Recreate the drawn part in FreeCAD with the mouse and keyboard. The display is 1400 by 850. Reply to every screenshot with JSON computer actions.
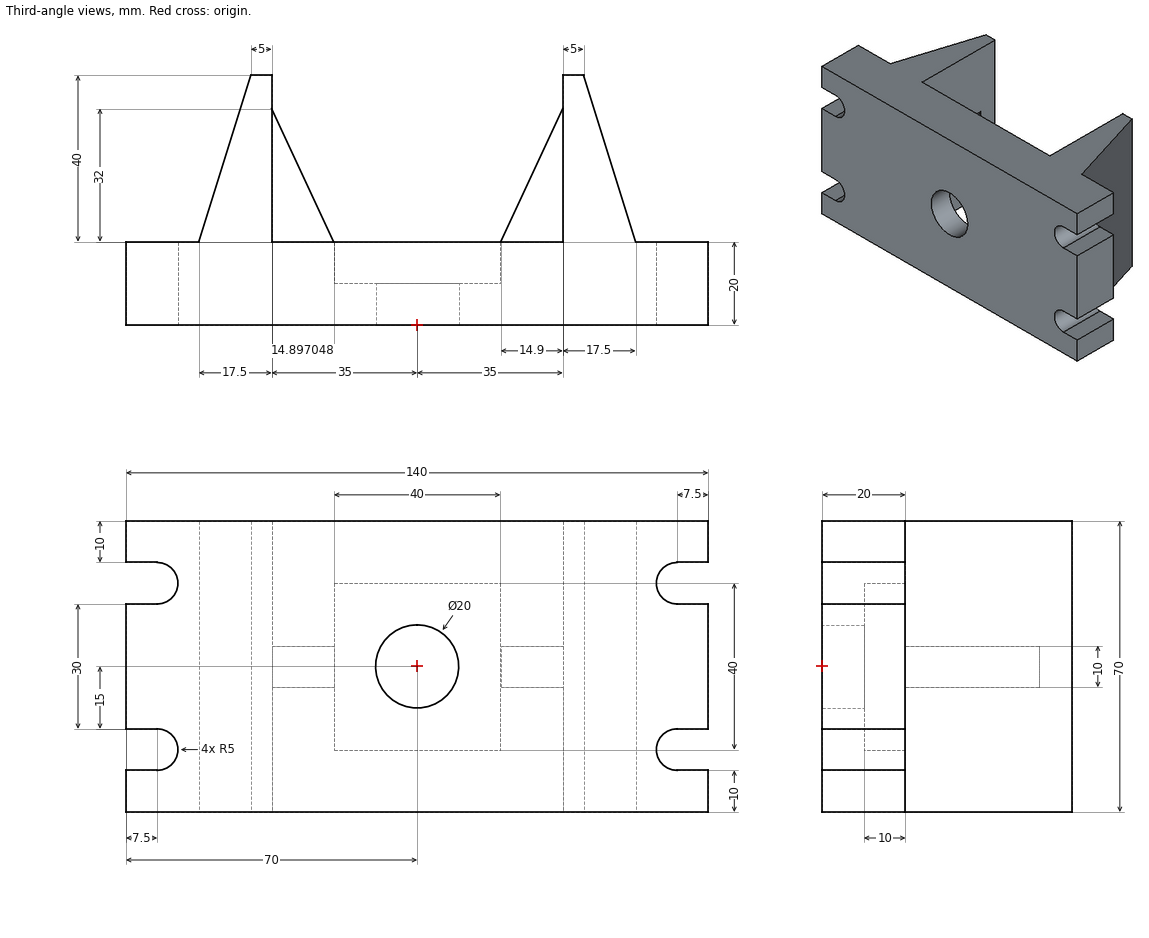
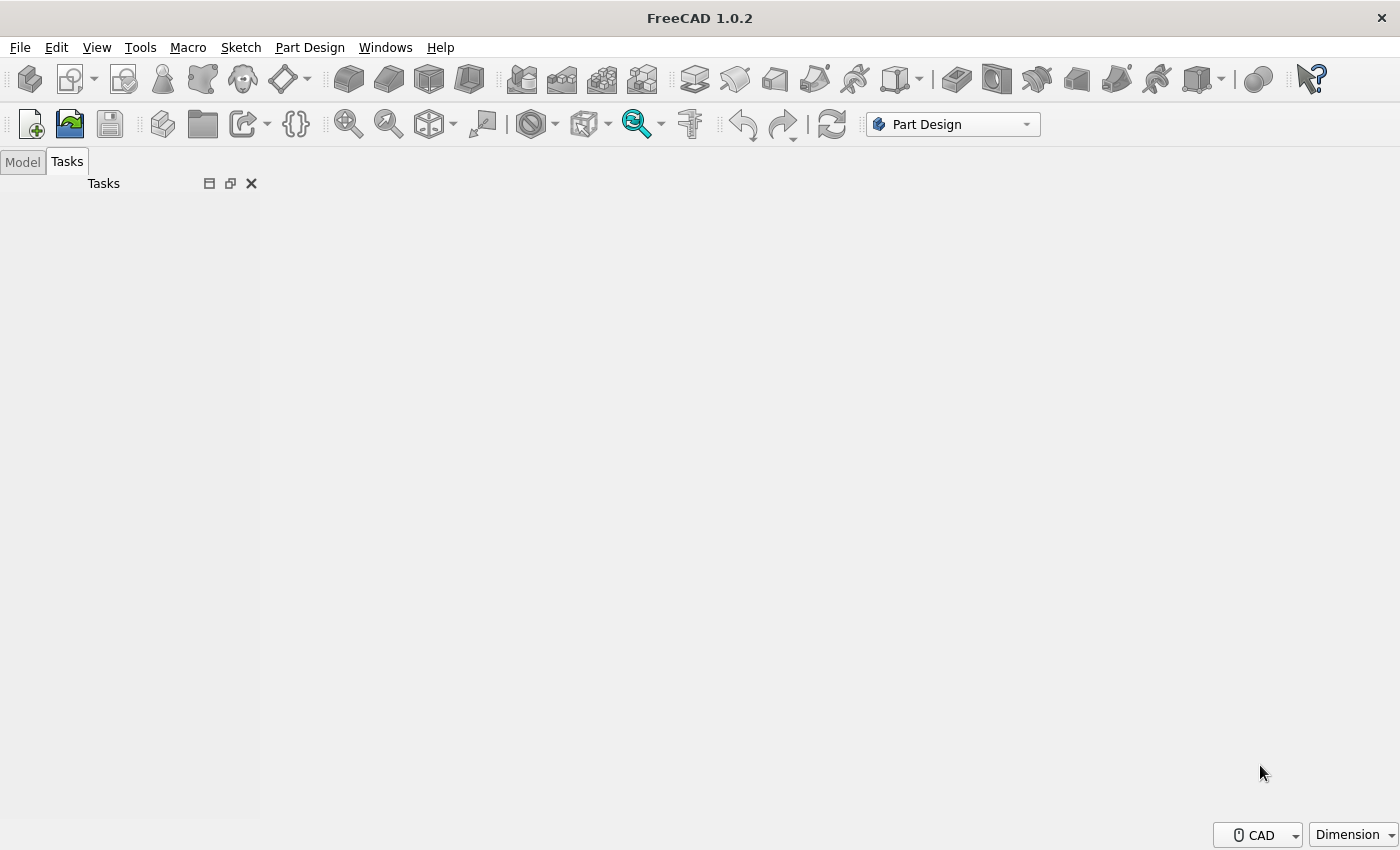
{"action": "left_click", "coordinate": [30, 124]}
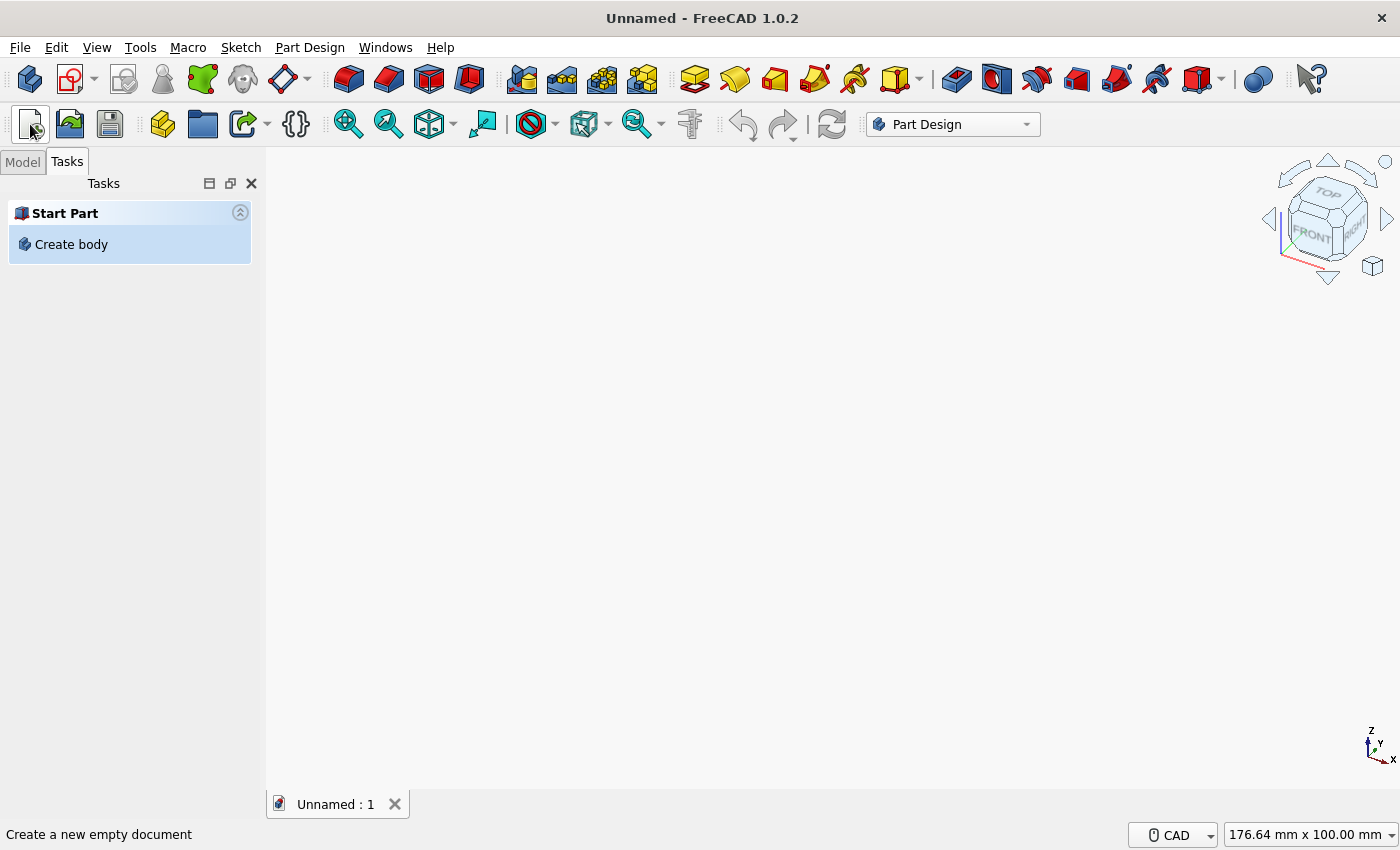
{"action": "left_click", "coordinate": [70, 80]}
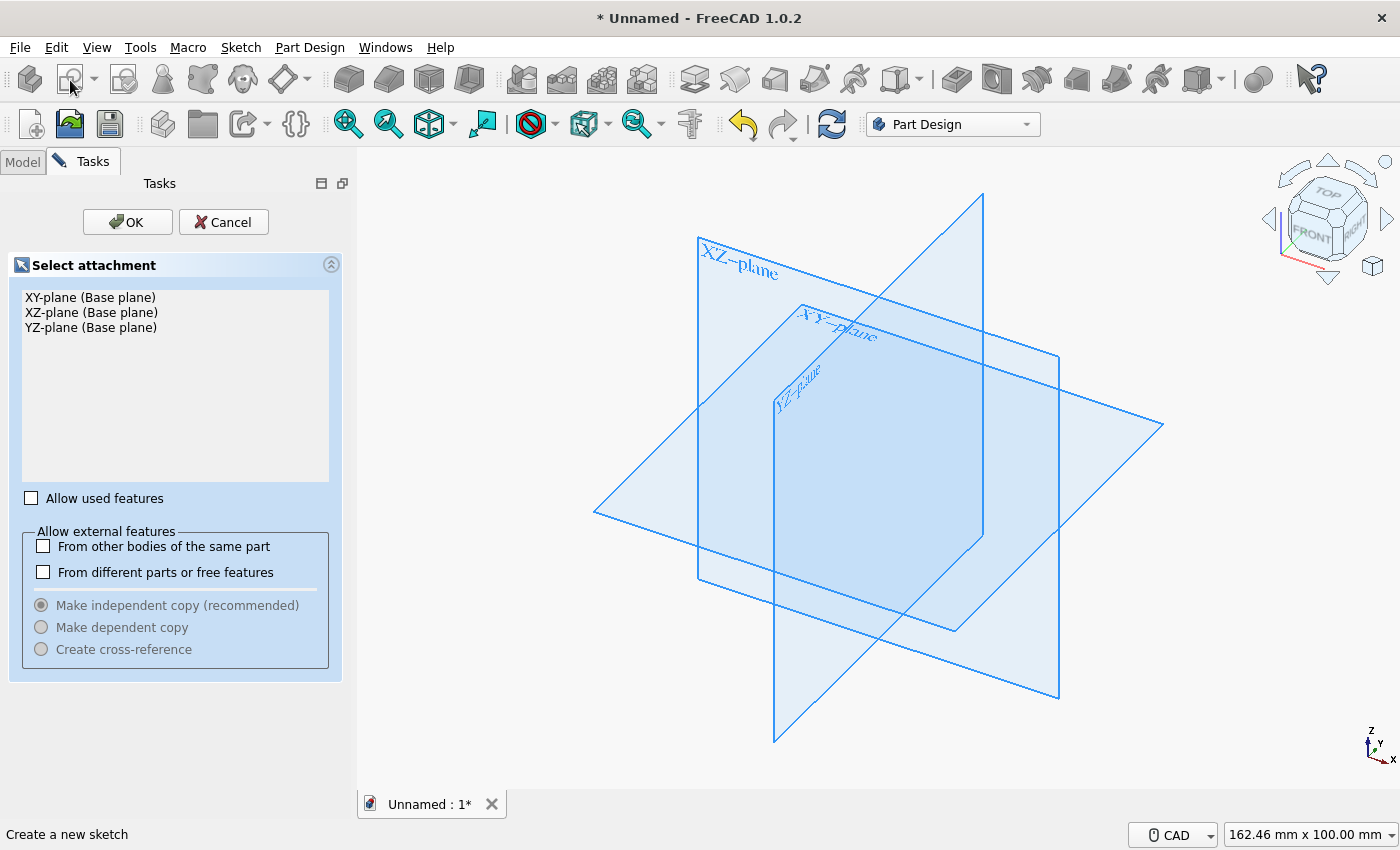
{"action": "left_click", "coordinate": [82, 312]}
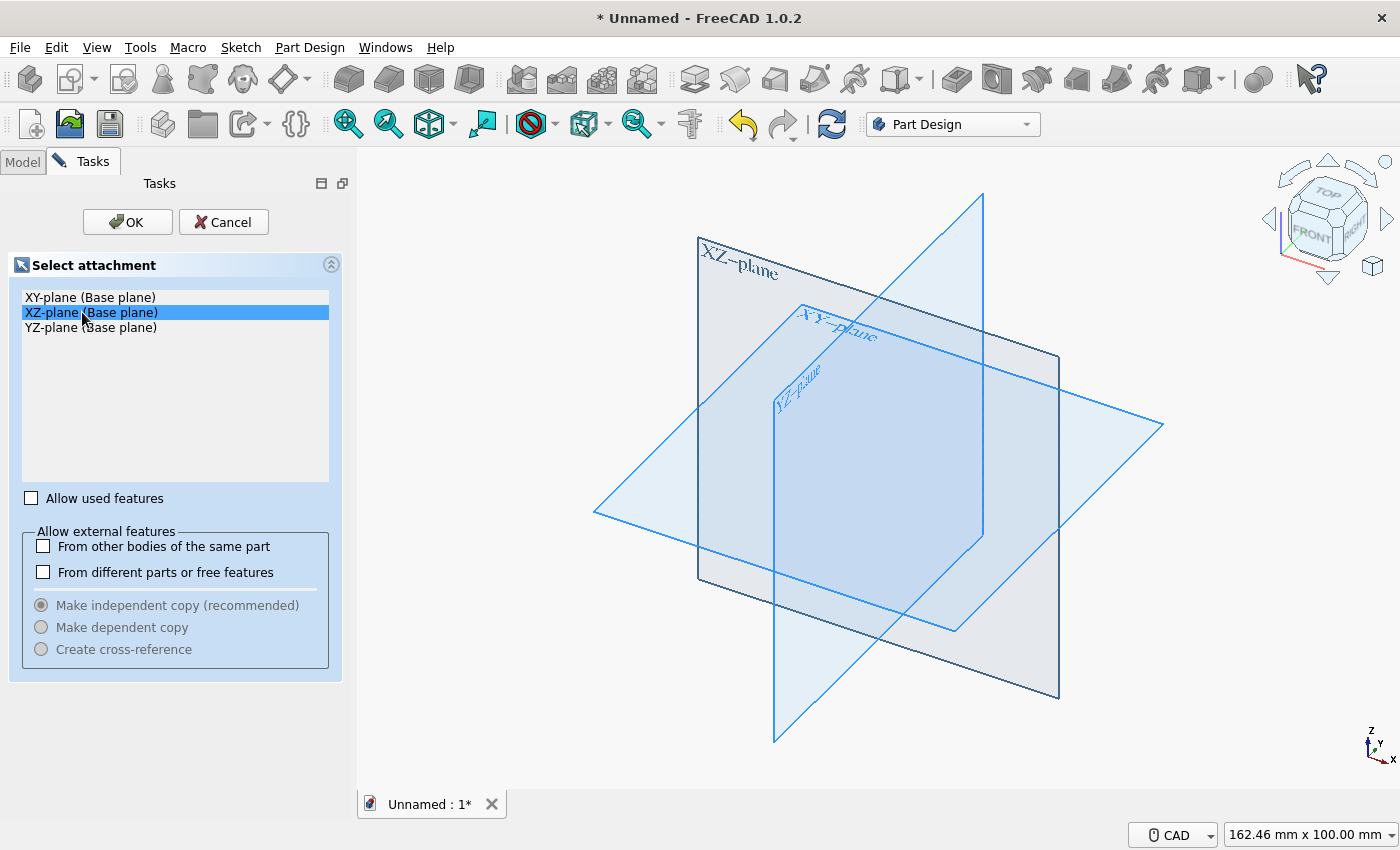
{"action": "left_click", "coordinate": [128, 222]}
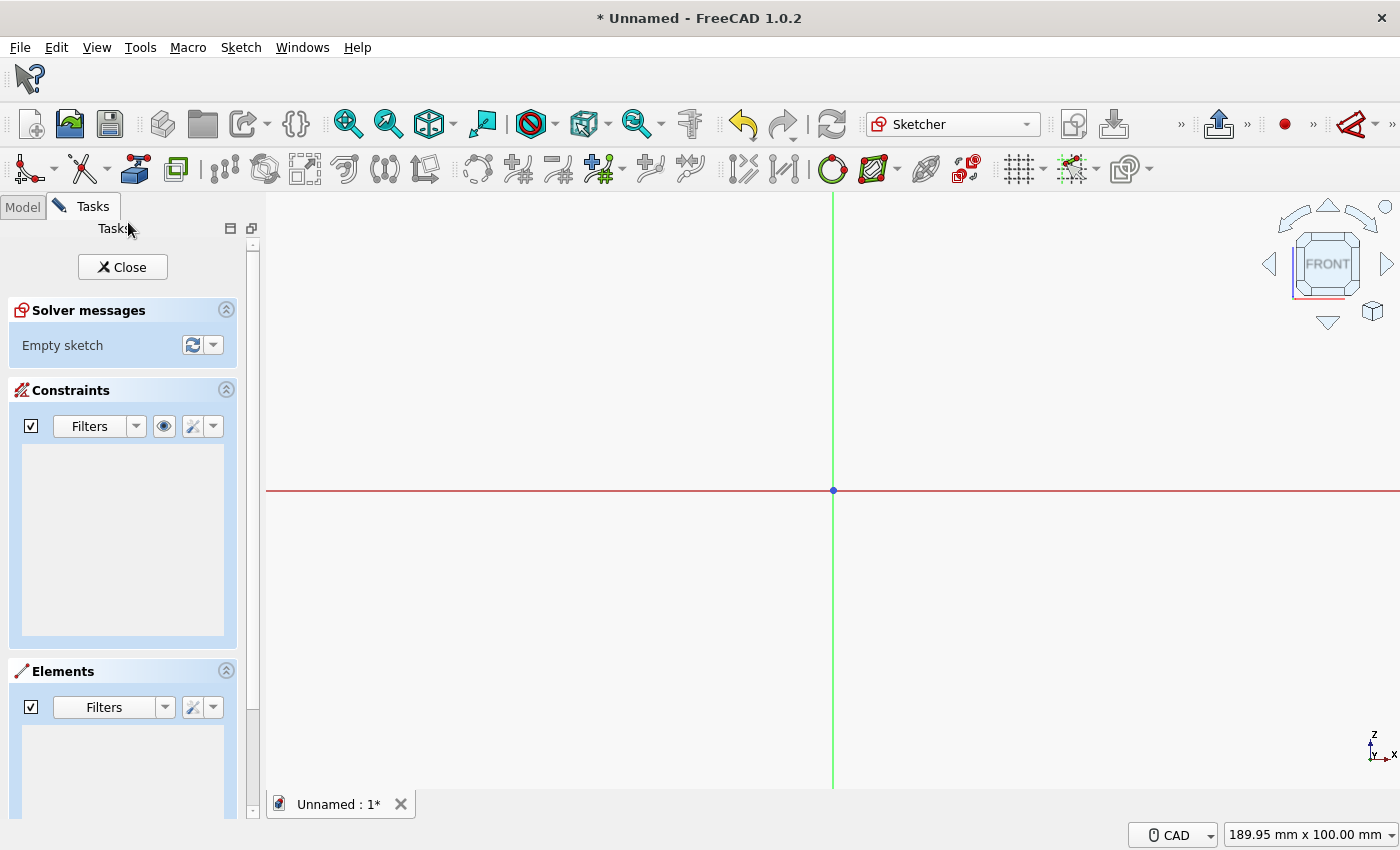
{"action": "scroll", "coordinate": [455, 490], "scroll_direction": "down", "scroll_amount": 1}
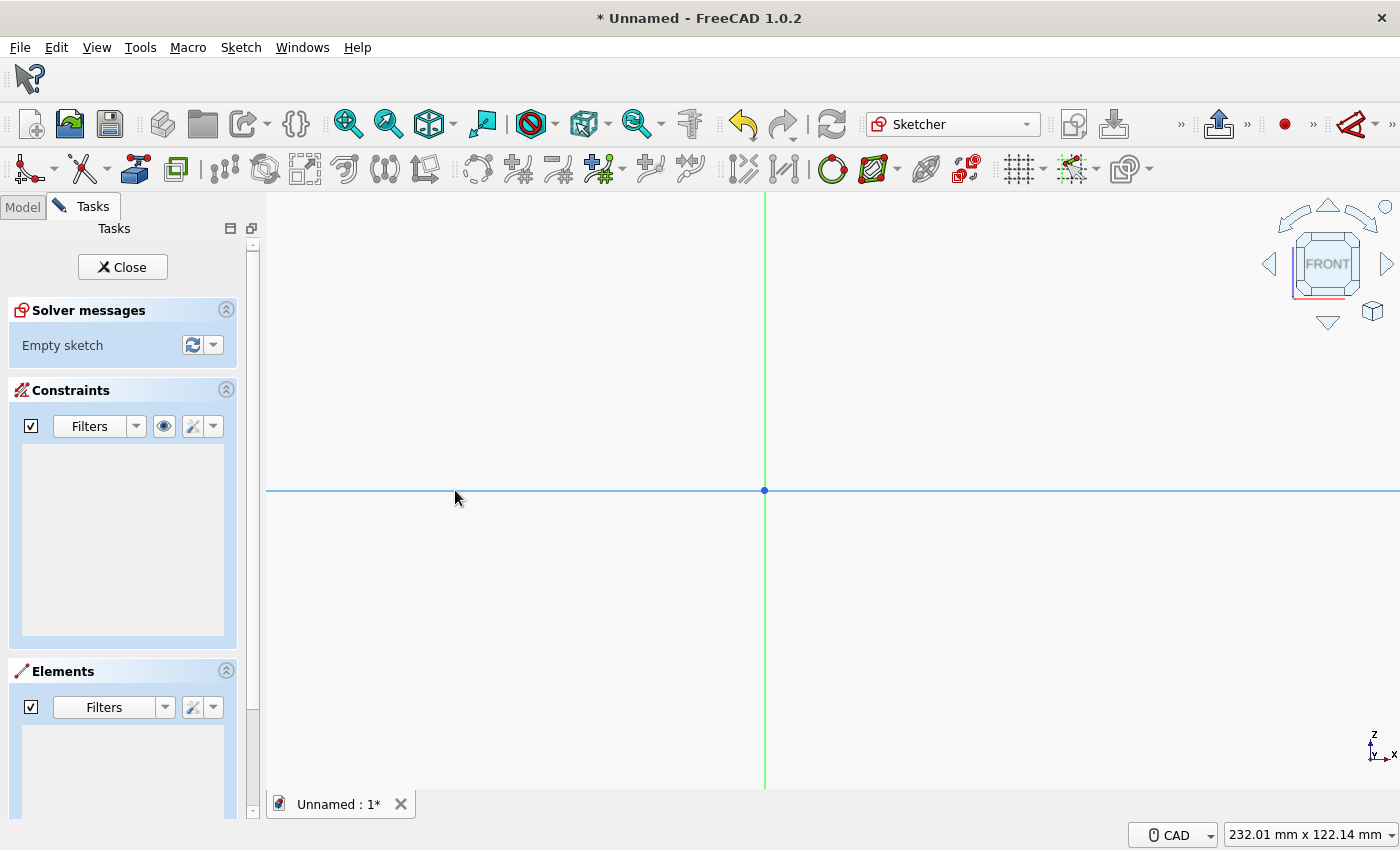
{"action": "key", "text": "g m"}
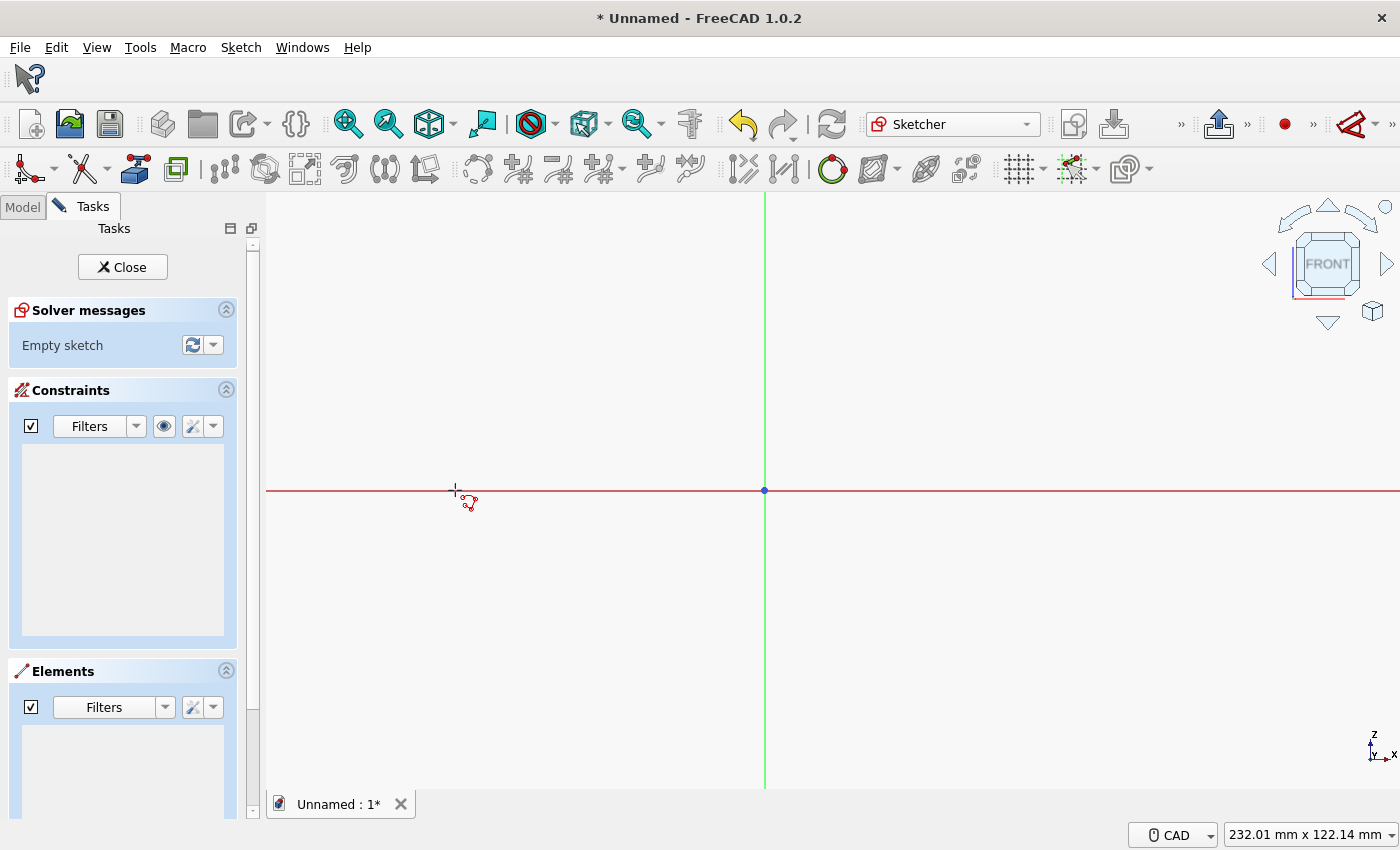
{"action": "left_click", "coordinate": [459, 564]}
{"action": "left_click", "coordinate": [422, 564]}
{"action": "left_click", "coordinate": [422, 417]}
{"action": "left_click", "coordinate": [459, 417]}
{"action": "right_click", "coordinate": [459, 417]}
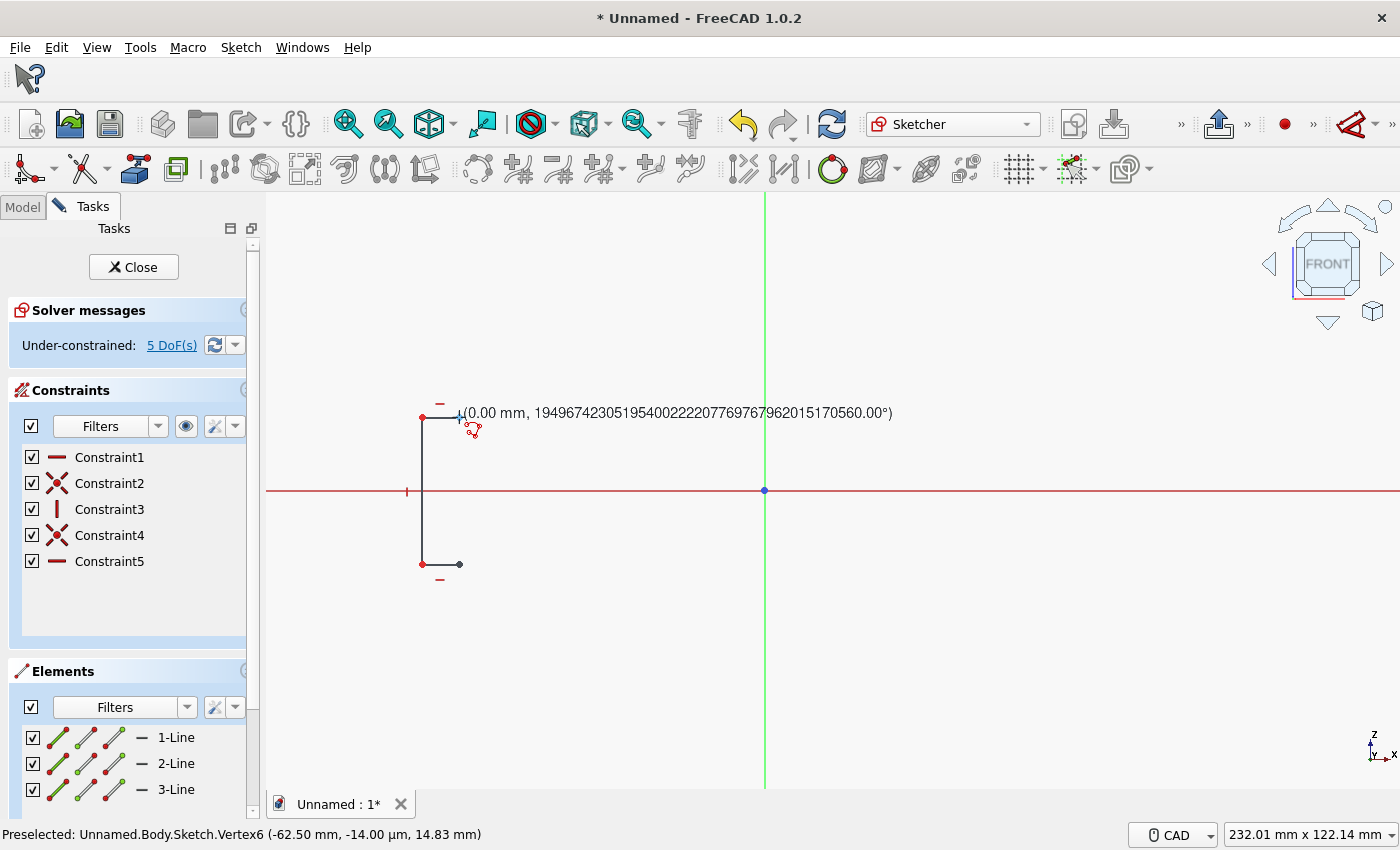
{"action": "left_click", "coordinate": [459, 368]}
{"action": "left_click", "coordinate": [422, 368]}
{"action": "left_click", "coordinate": [422, 319]}
{"action": "left_click", "coordinate": [1107, 319]}
{"action": "left_click", "coordinate": [1107, 368]}
{"action": "left_click", "coordinate": [1070, 368]}
{"action": "right_click", "coordinate": [1070, 368]}